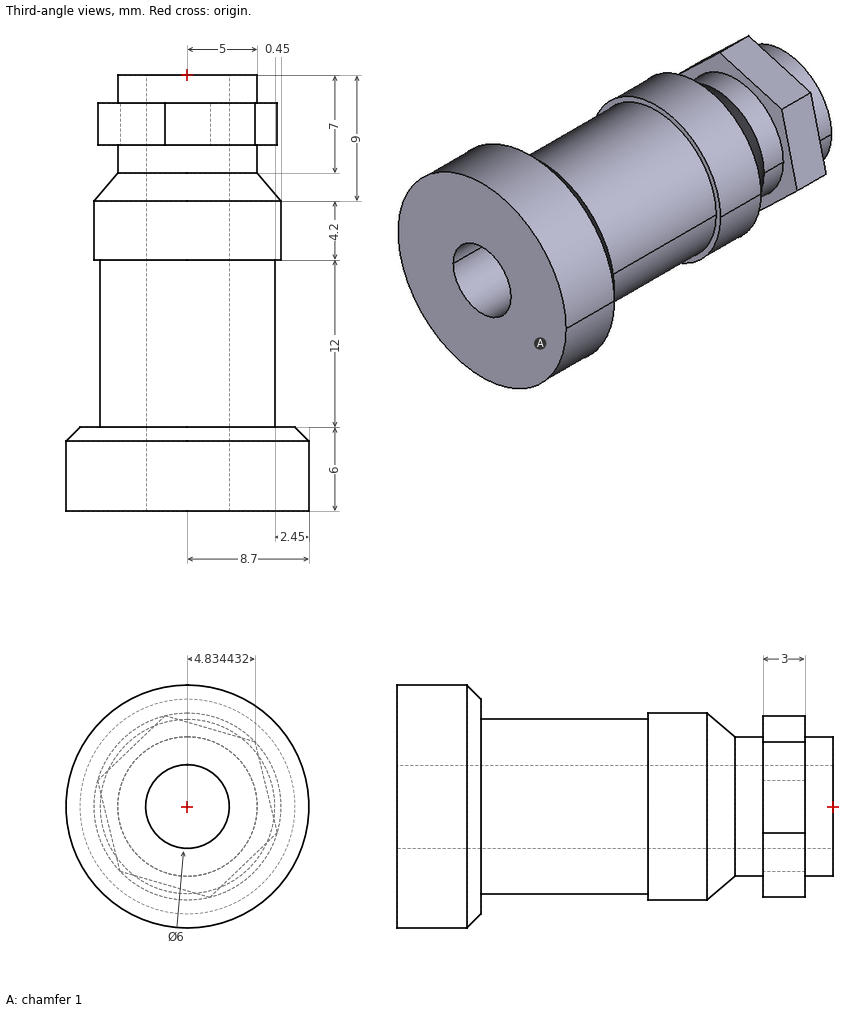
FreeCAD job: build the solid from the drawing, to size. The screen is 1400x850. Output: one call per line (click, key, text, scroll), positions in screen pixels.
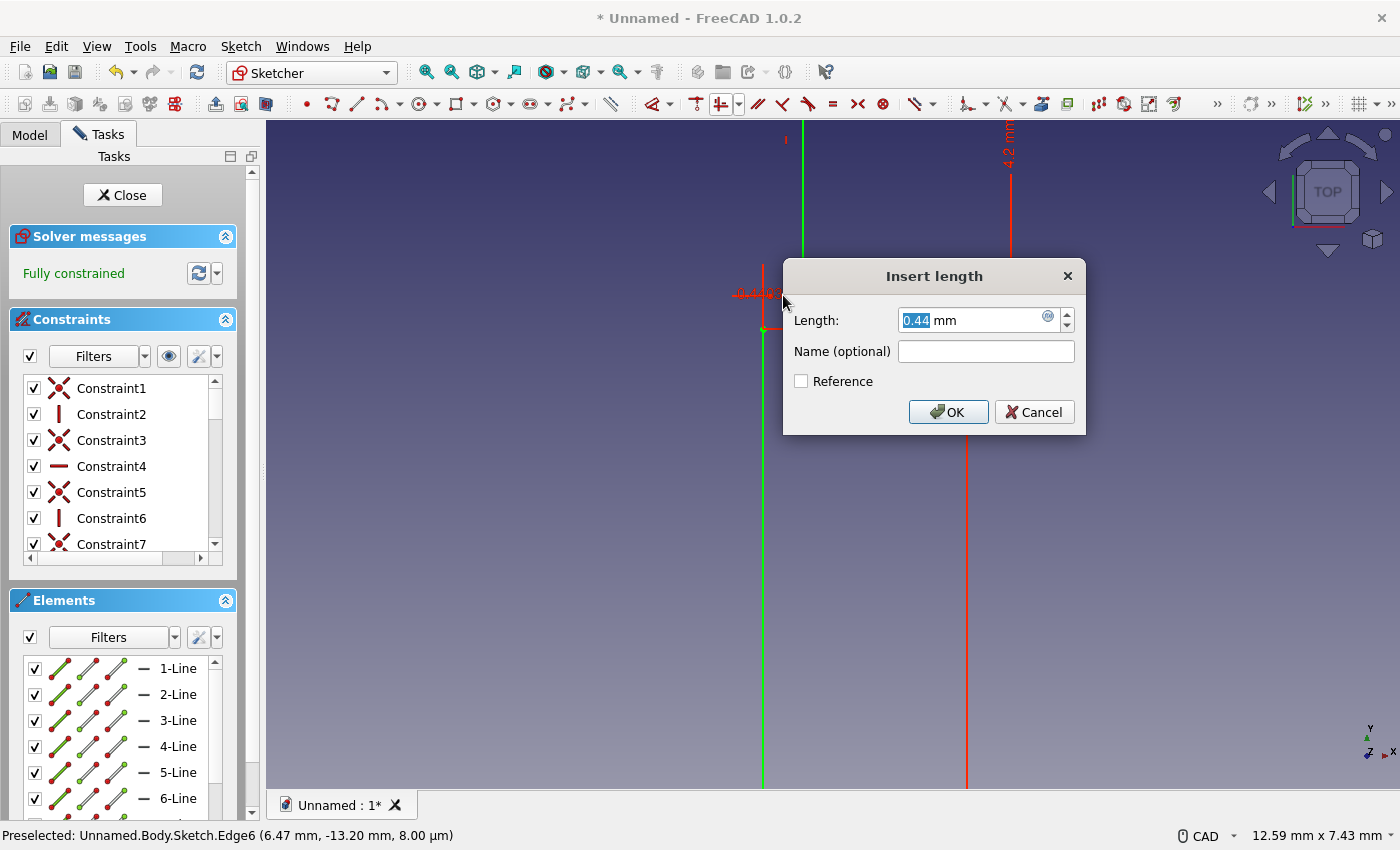
text(0.45)
key(Return)
key(Escape)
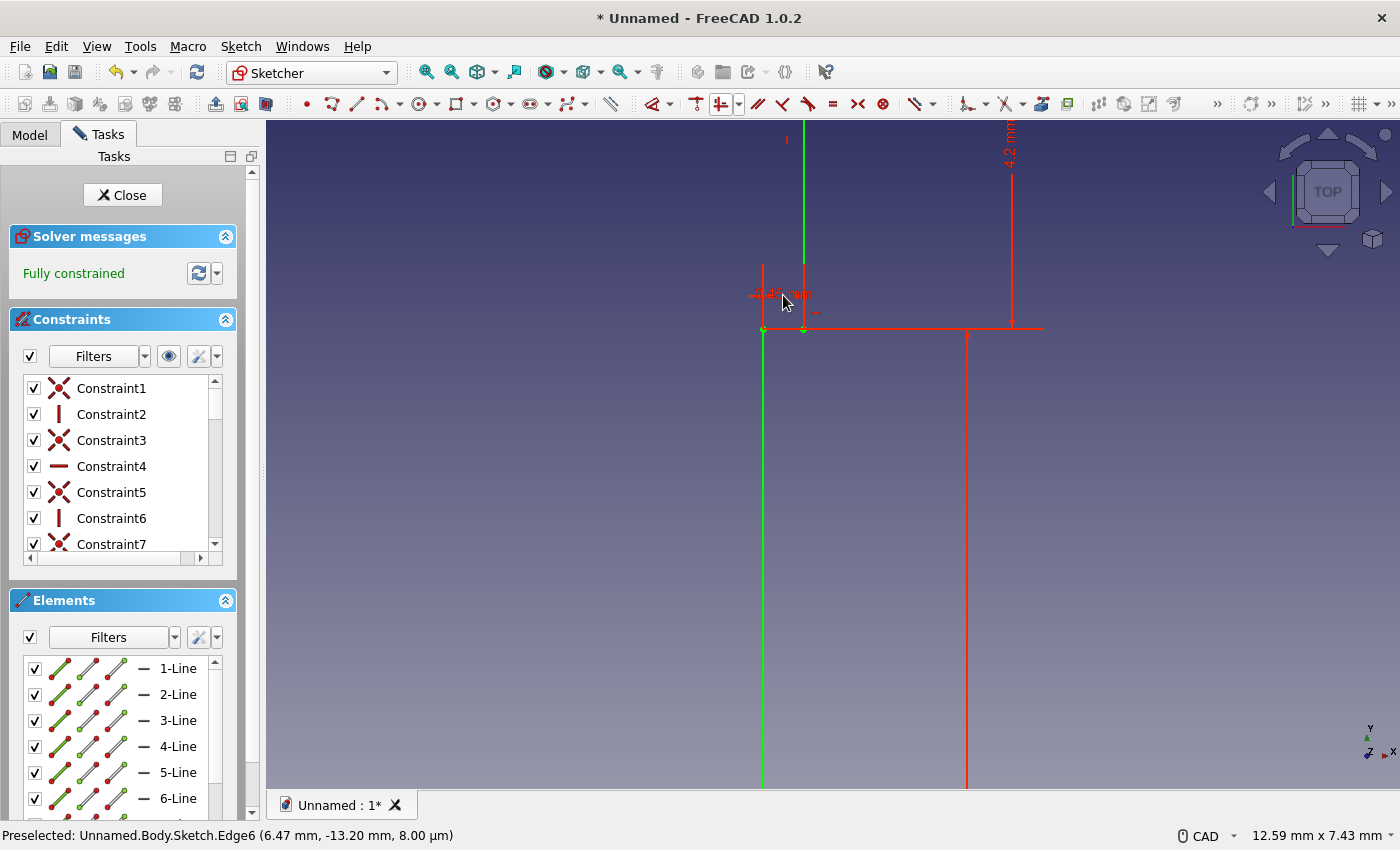
click(123, 195)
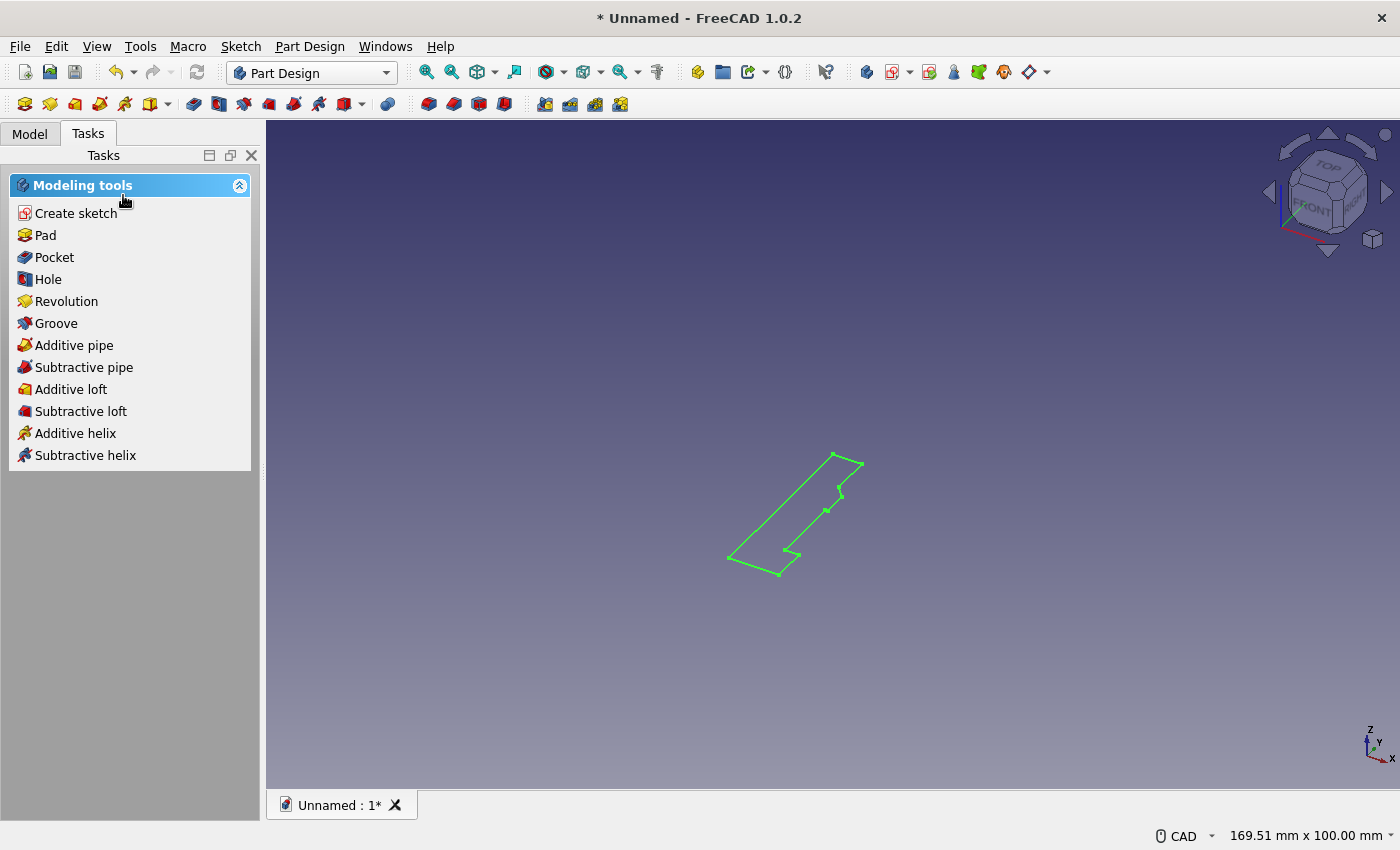
click(50, 104)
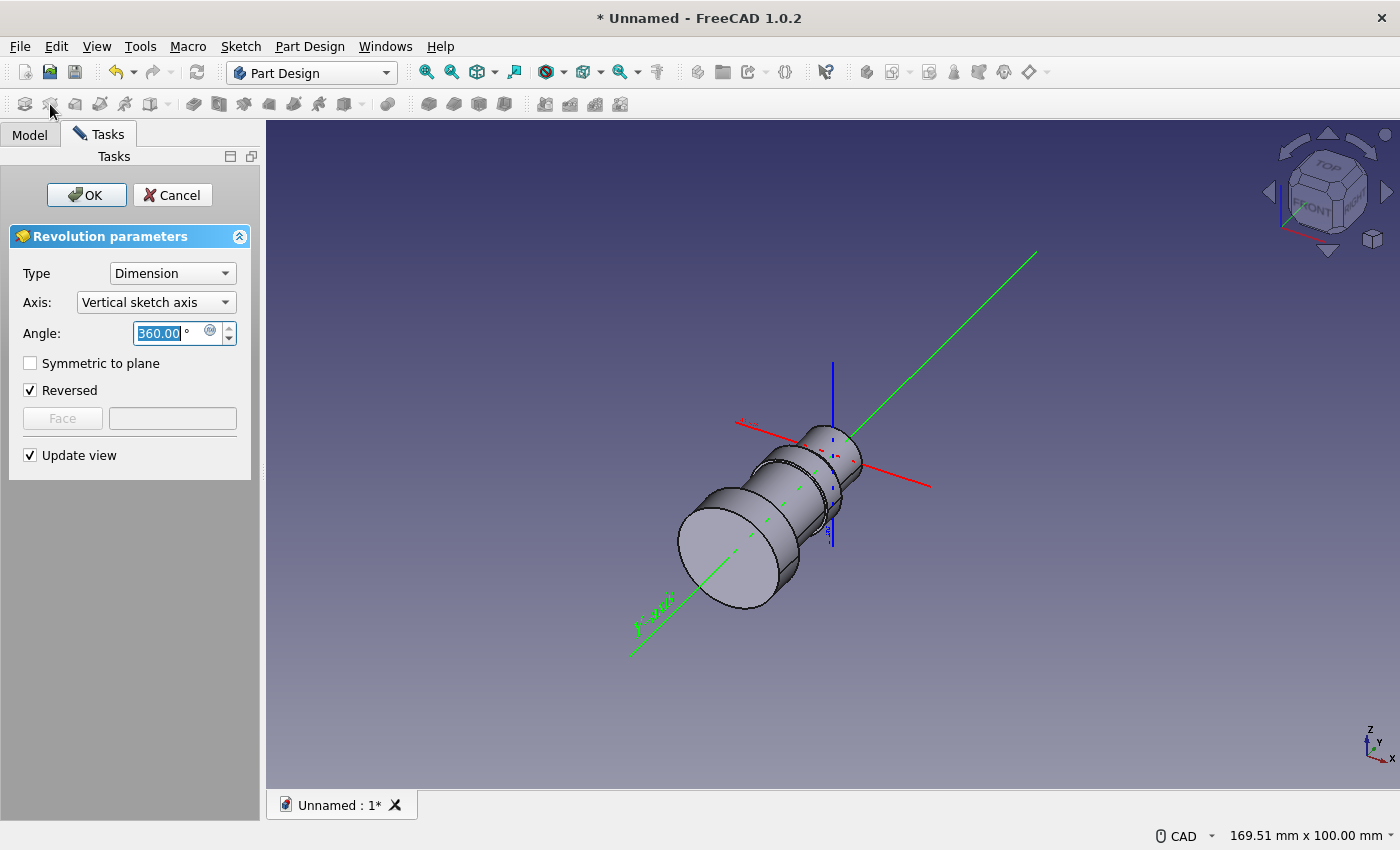
click(87, 195)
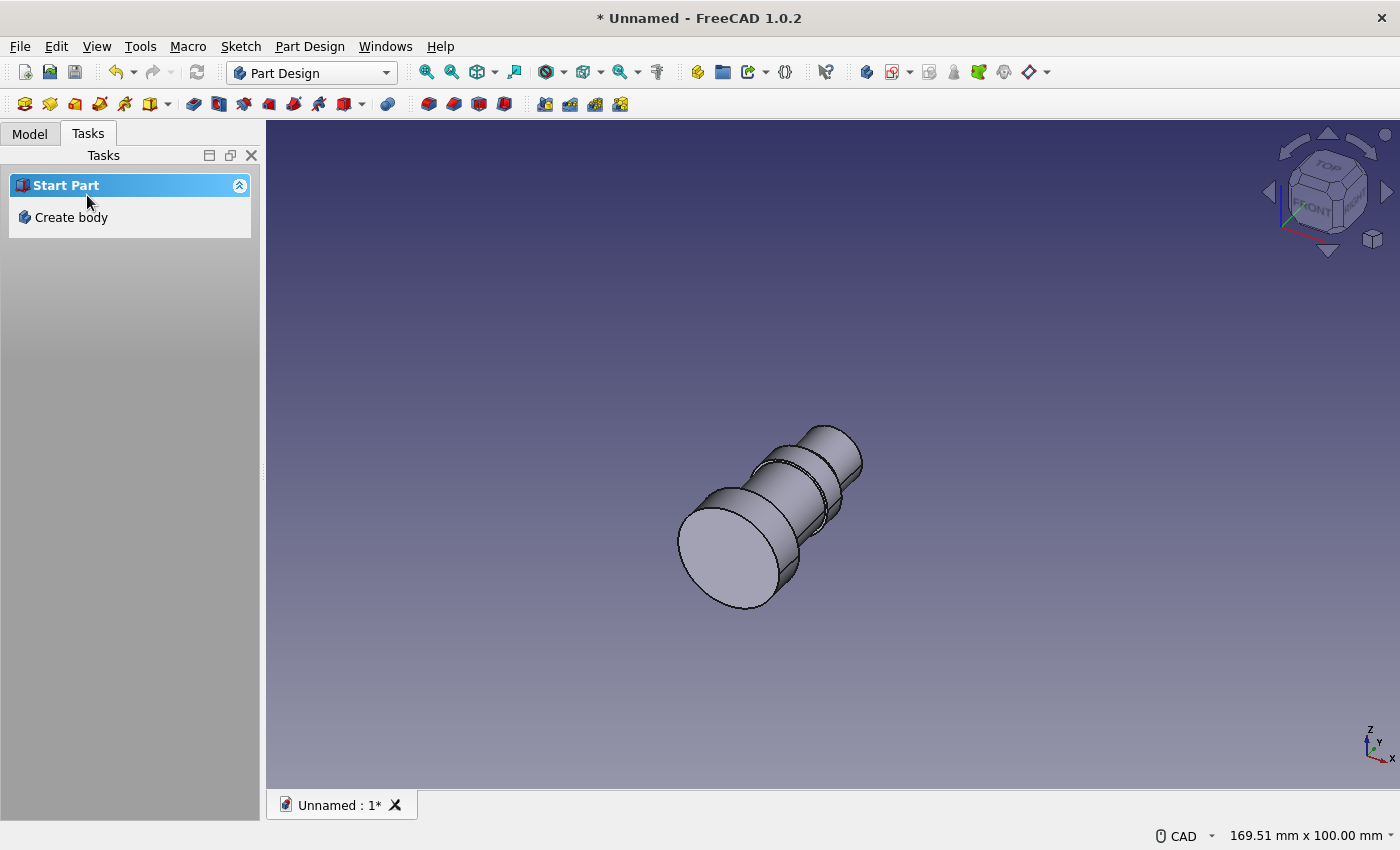
key(v)
key(f)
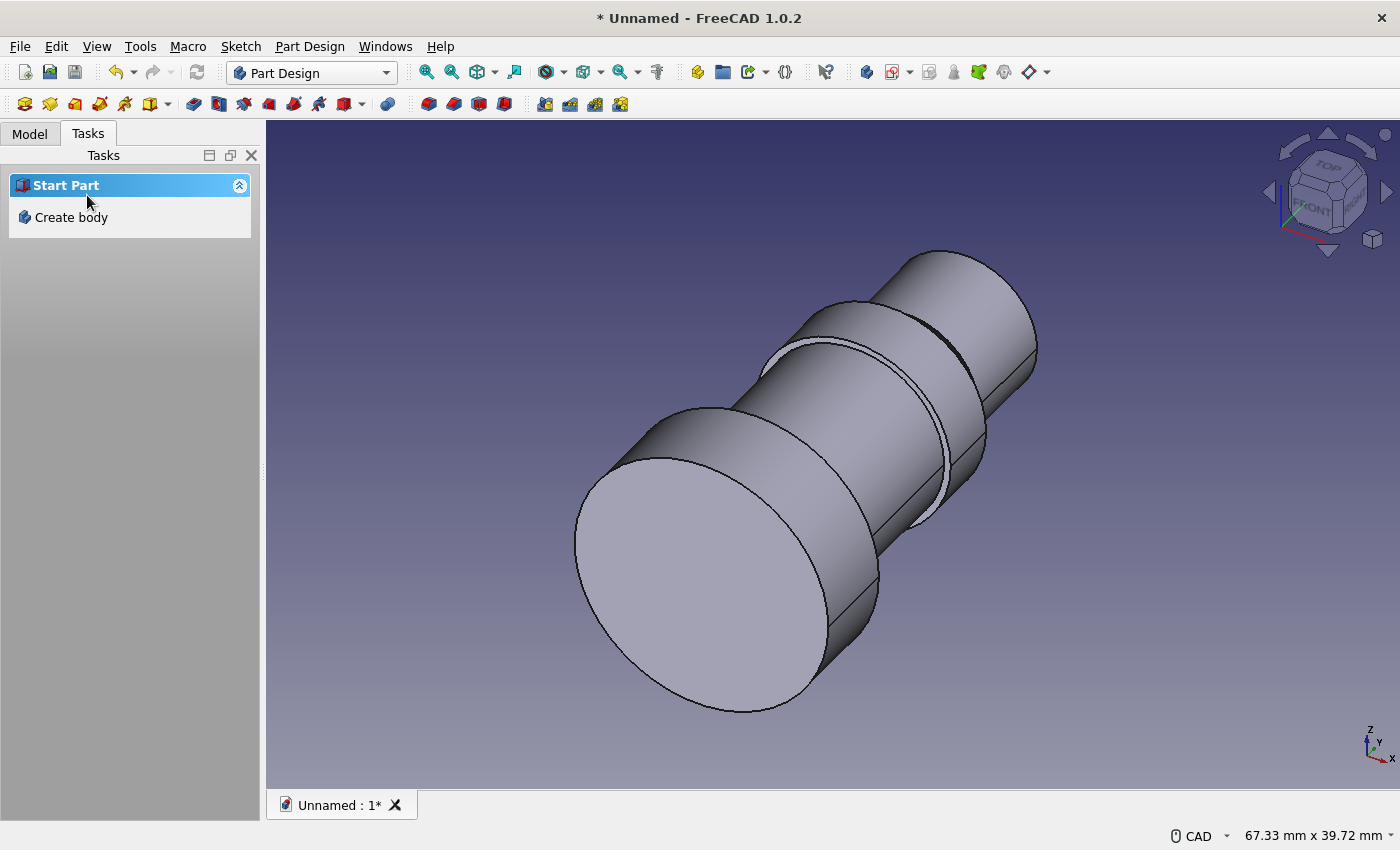
click(30, 134)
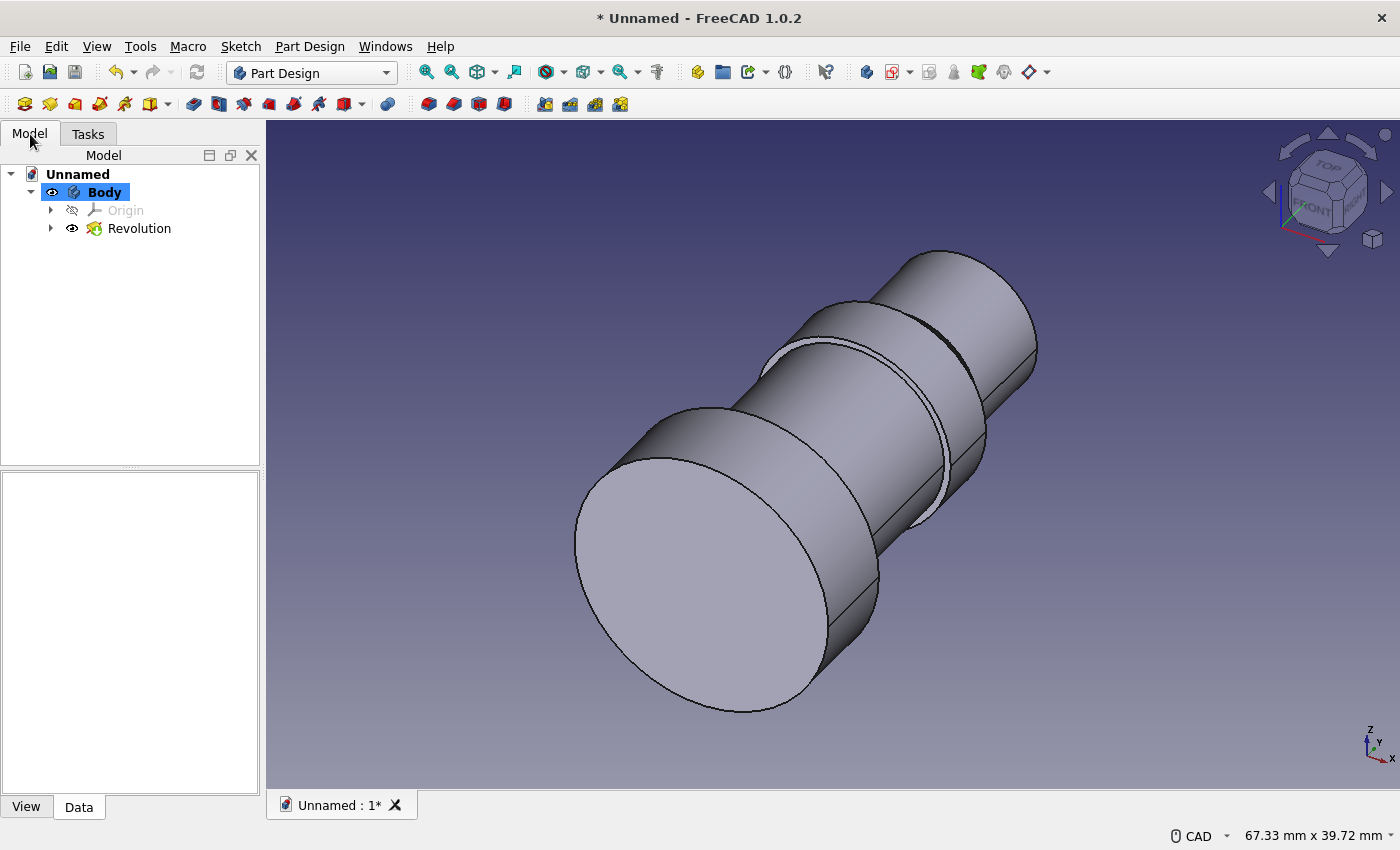
click(51, 210)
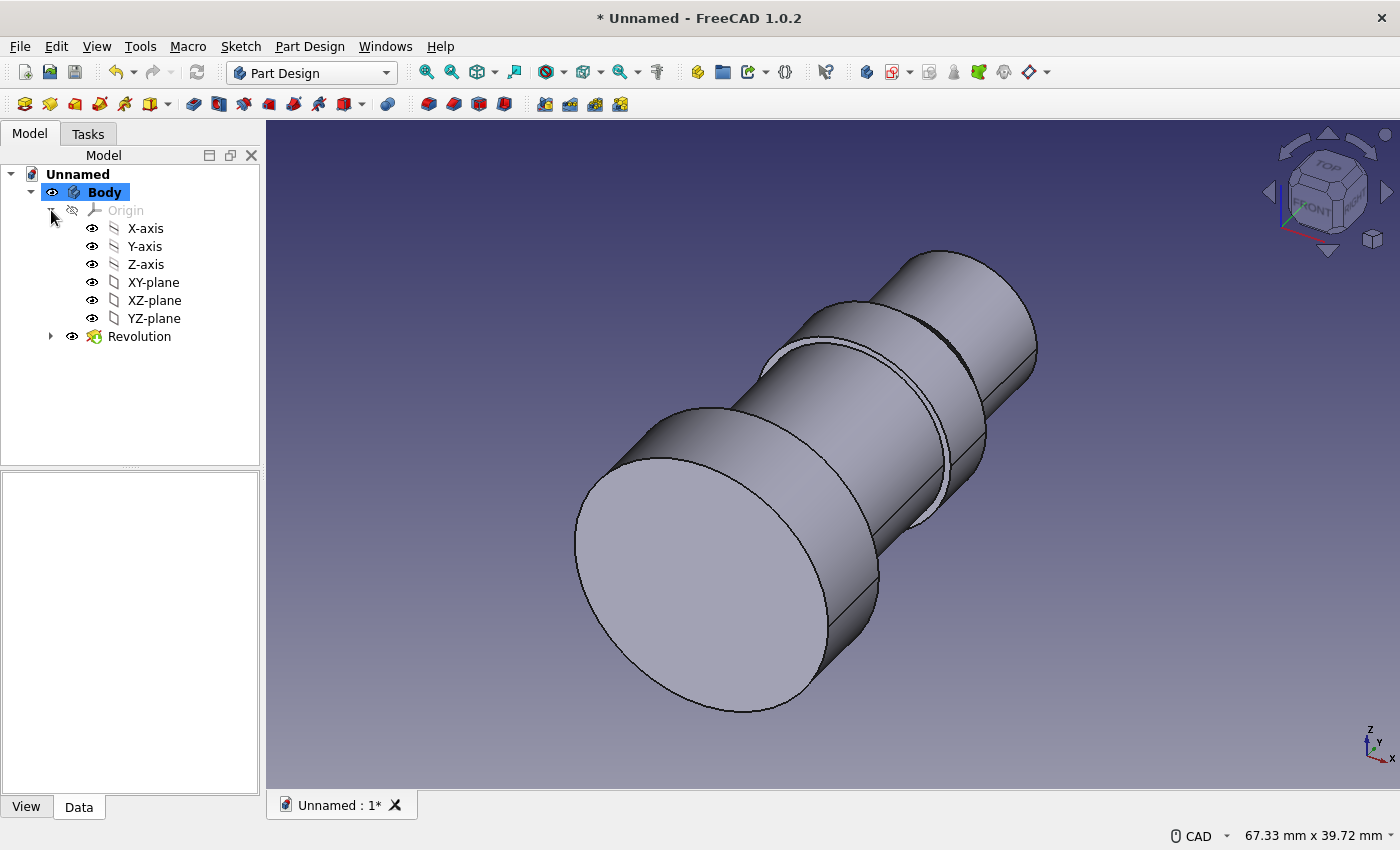
click(137, 300)